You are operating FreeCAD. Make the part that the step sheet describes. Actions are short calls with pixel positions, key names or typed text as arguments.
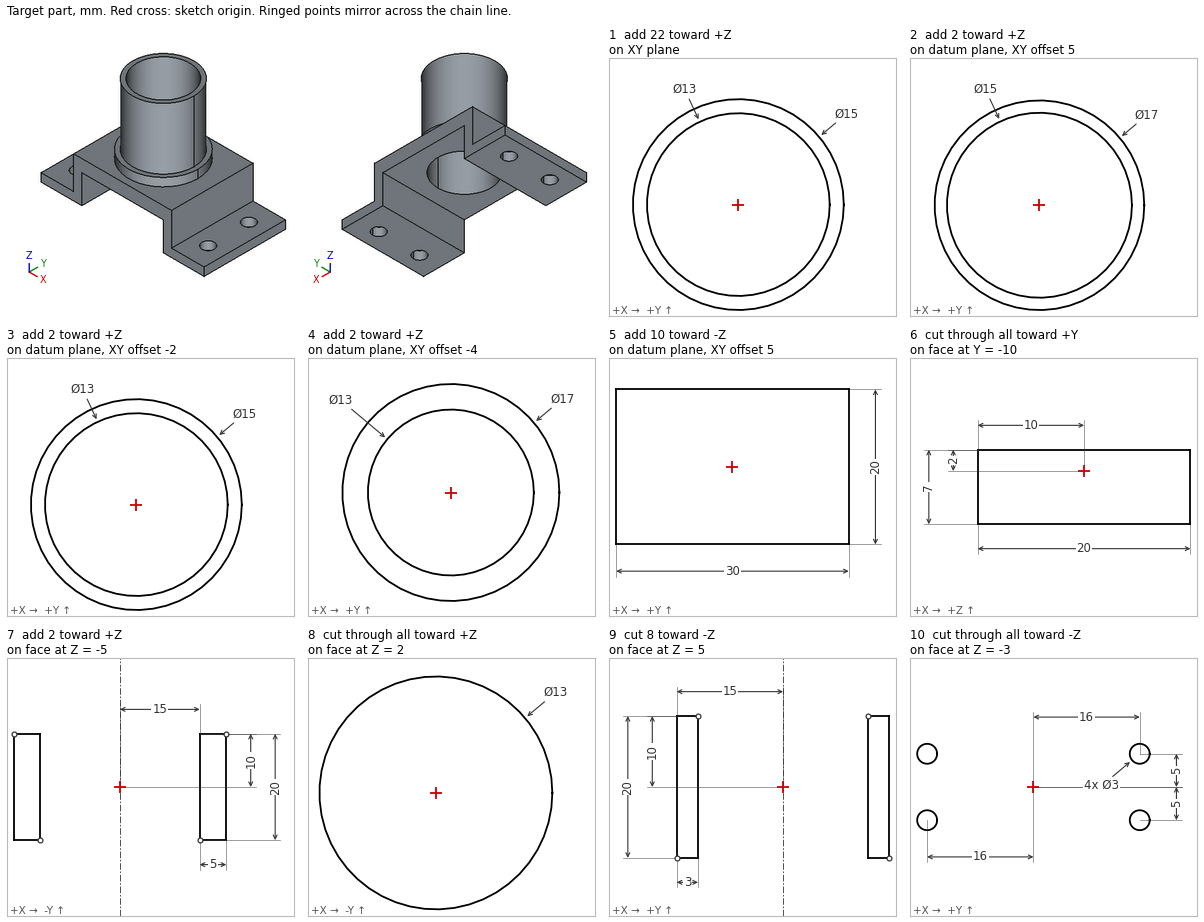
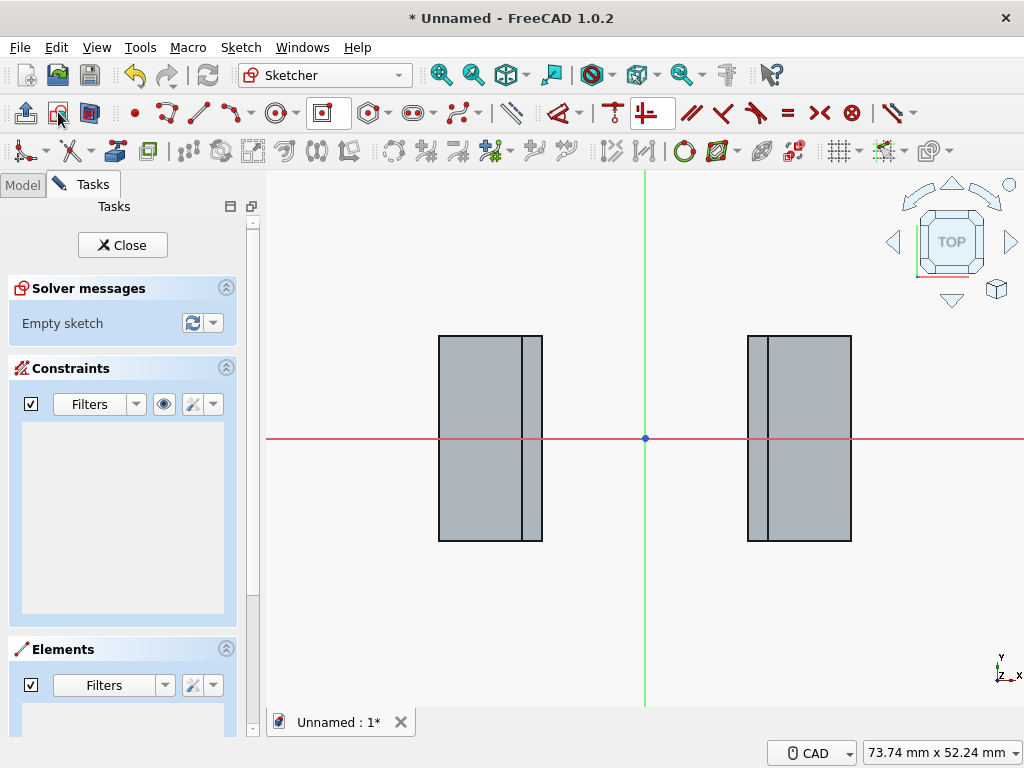
click(276, 114)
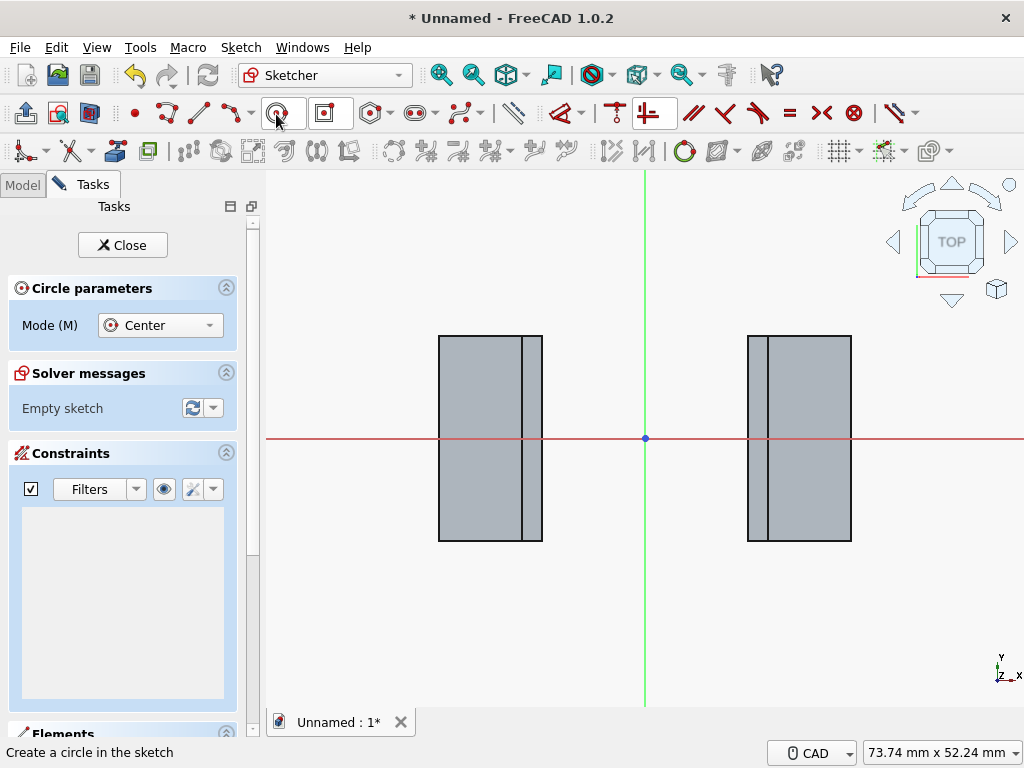
scroll(809, 387, up, 2)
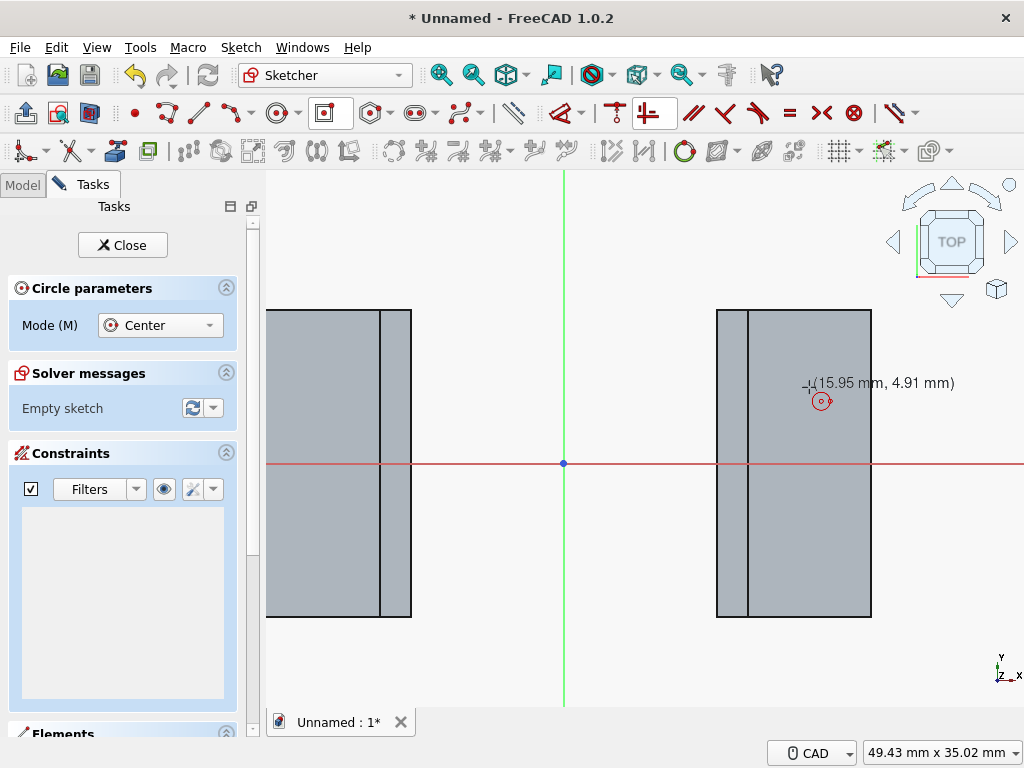
click(809, 387)
click(826, 371)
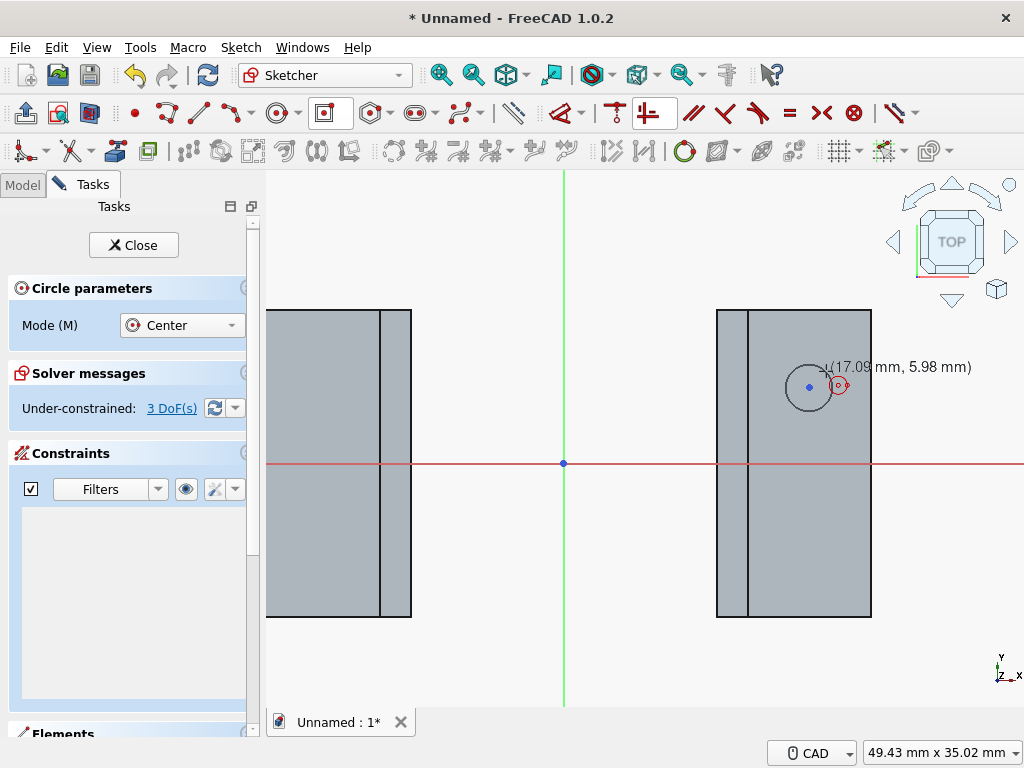
click(809, 540)
click(826, 524)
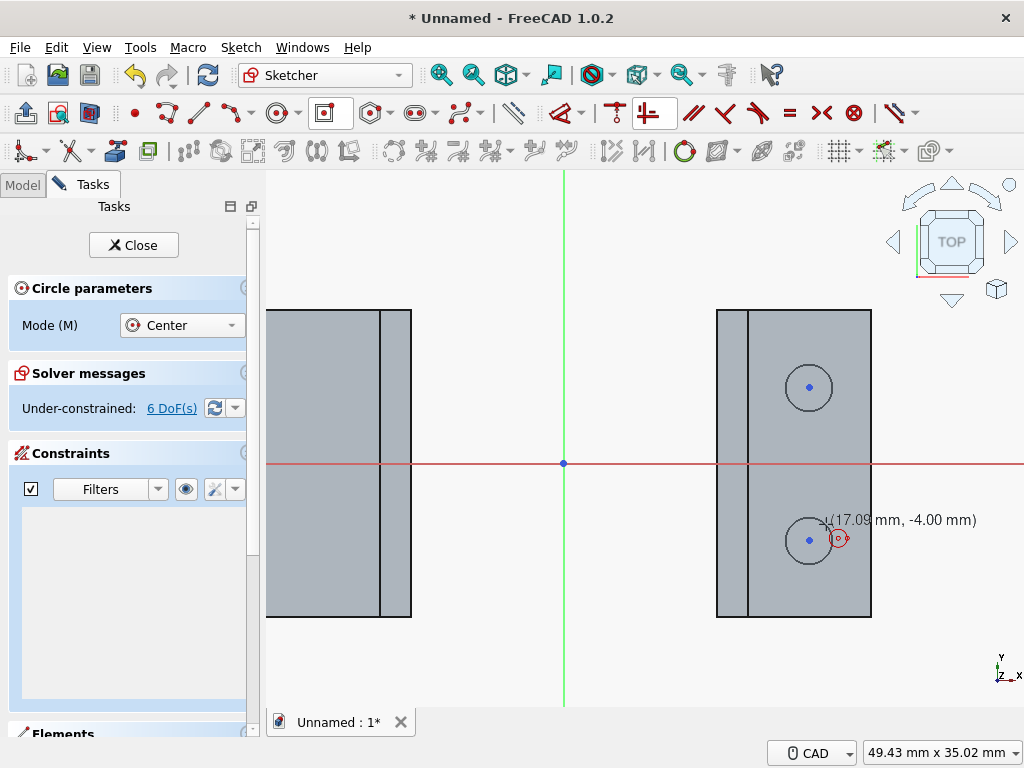
click(319, 540)
click(335, 524)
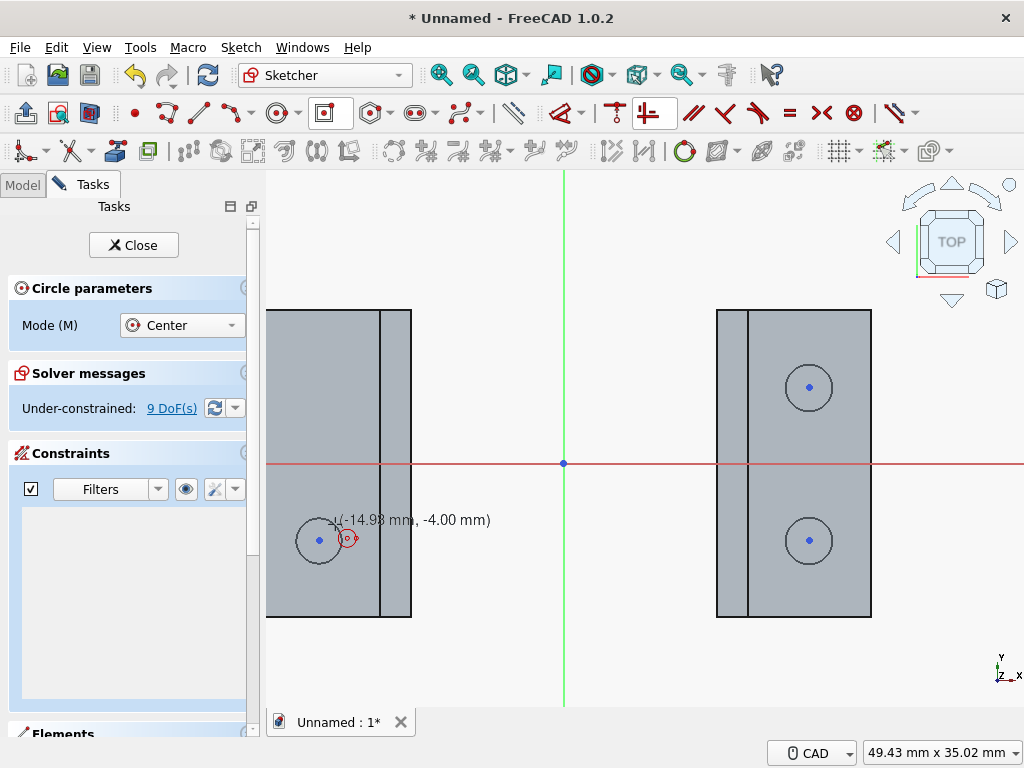
click(319, 387)
click(335, 371)
key(Escape)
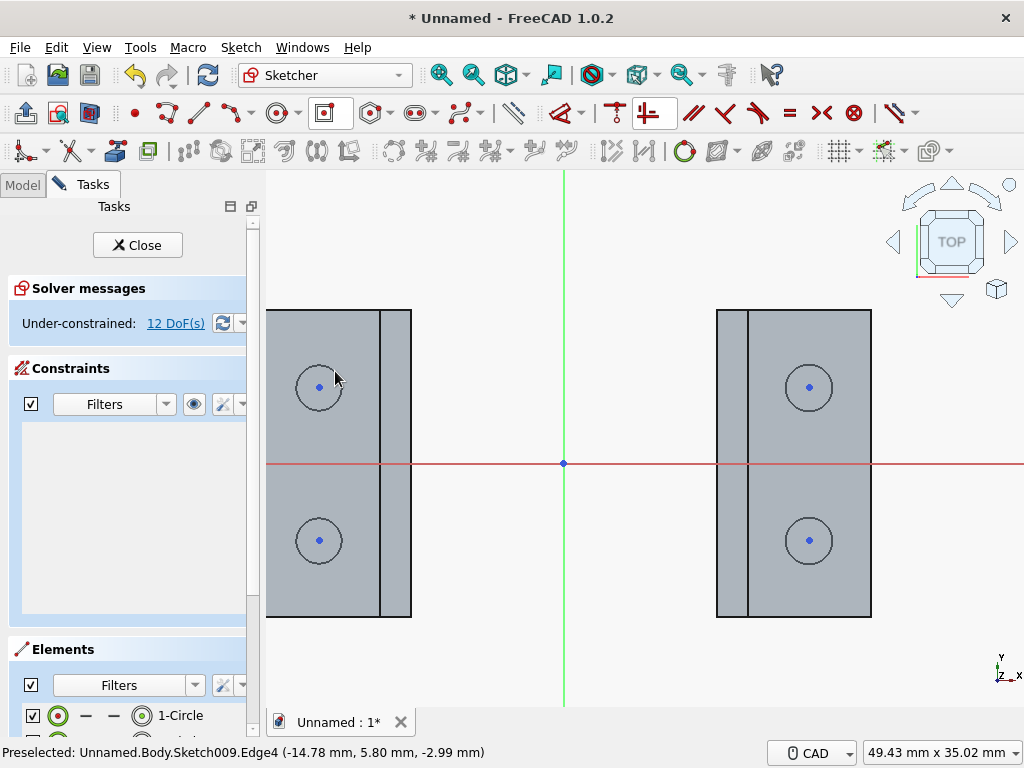
click(825, 371)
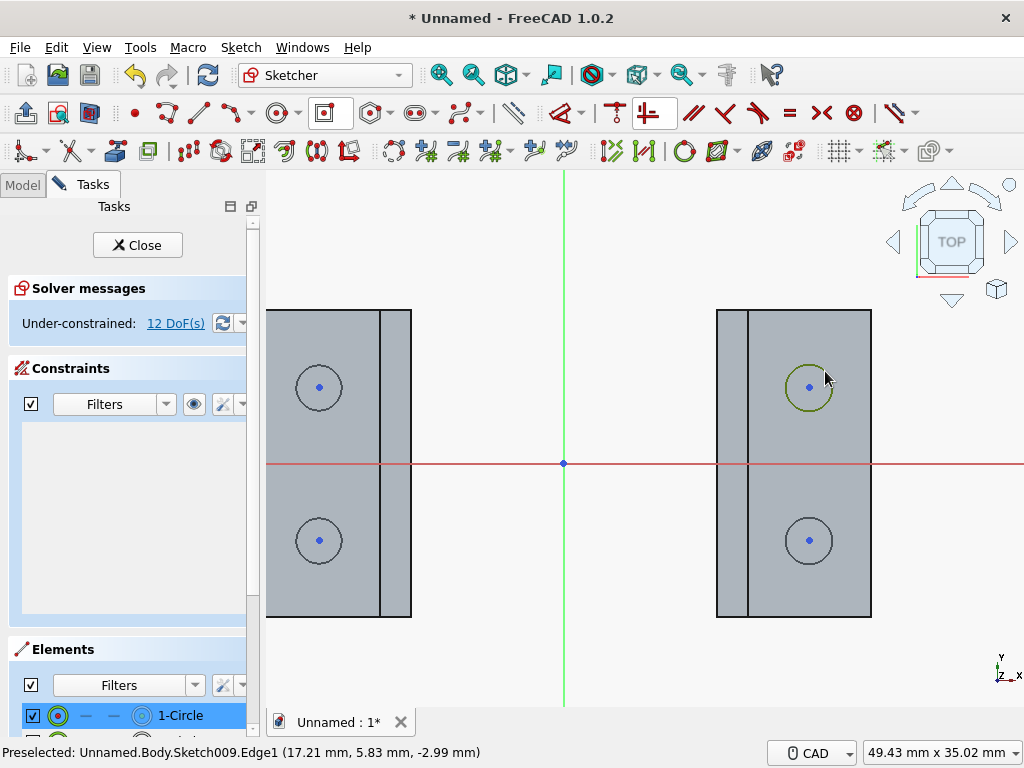
click(825, 524)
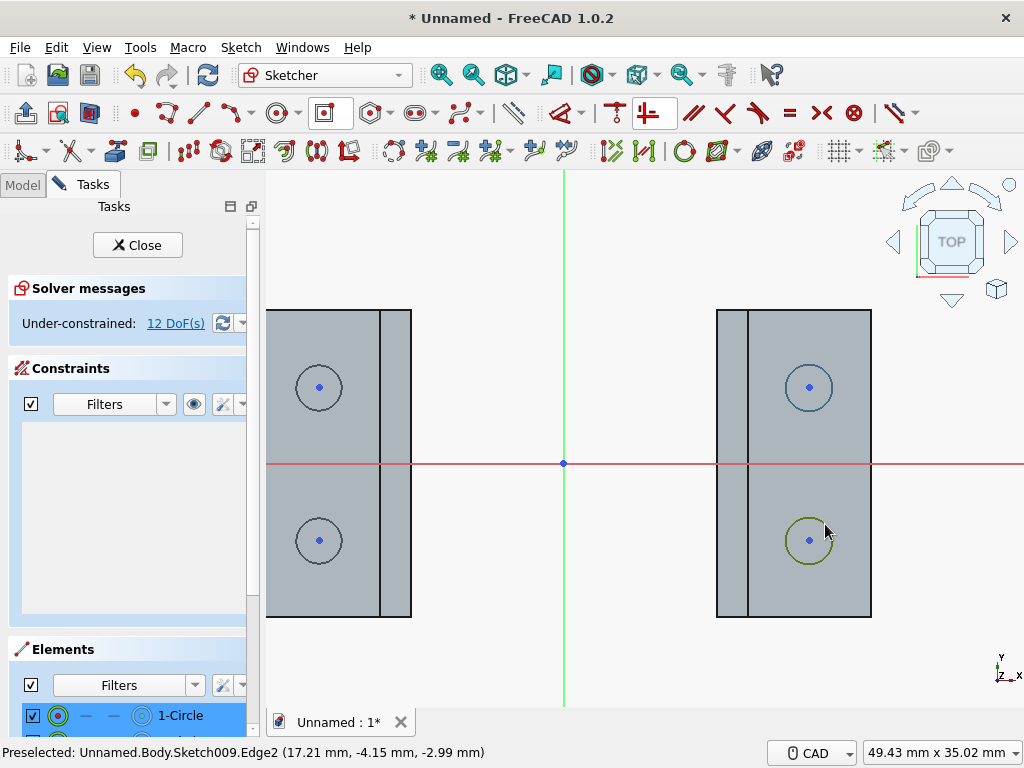
click(335, 525)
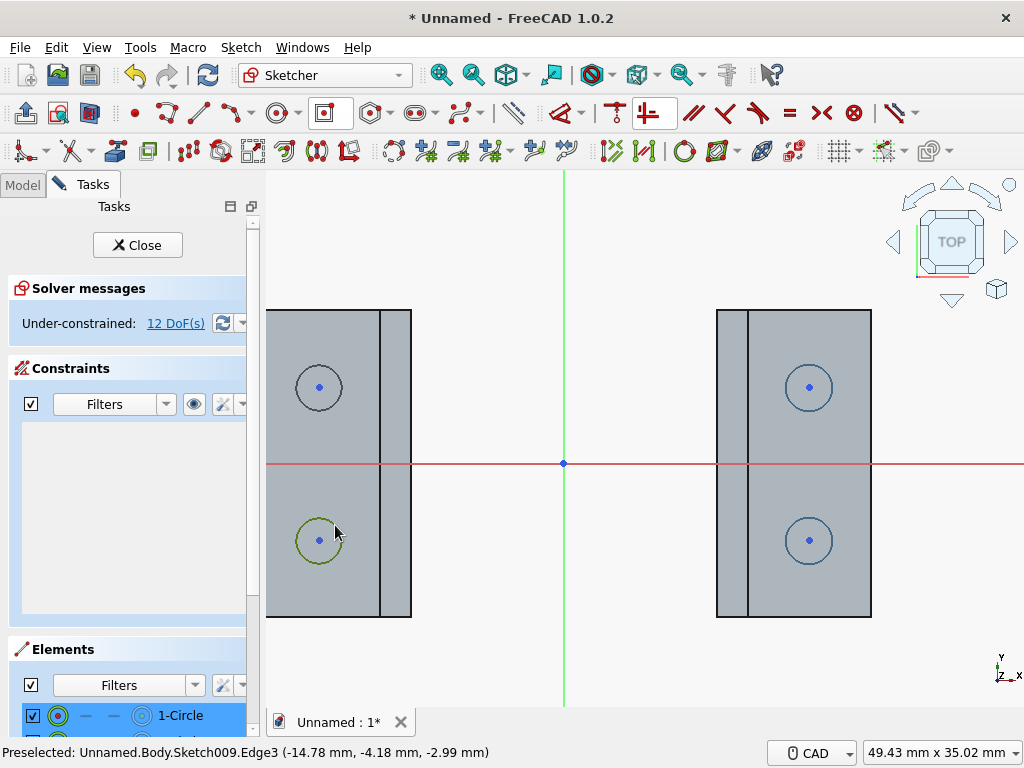
click(335, 372)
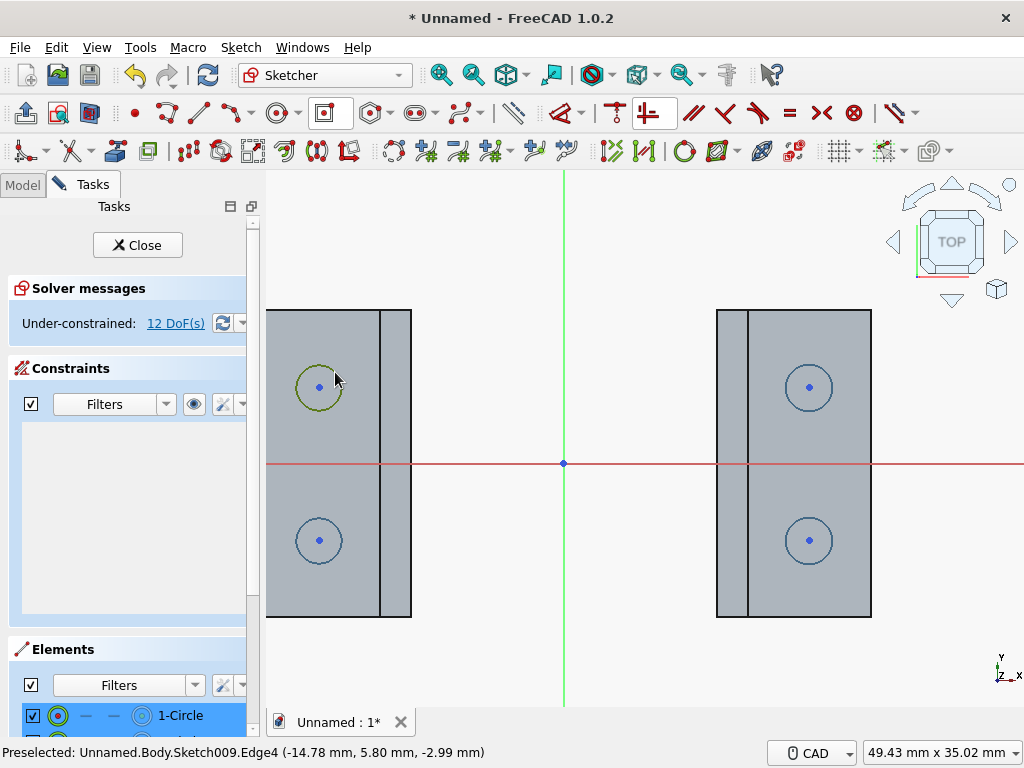
click(790, 114)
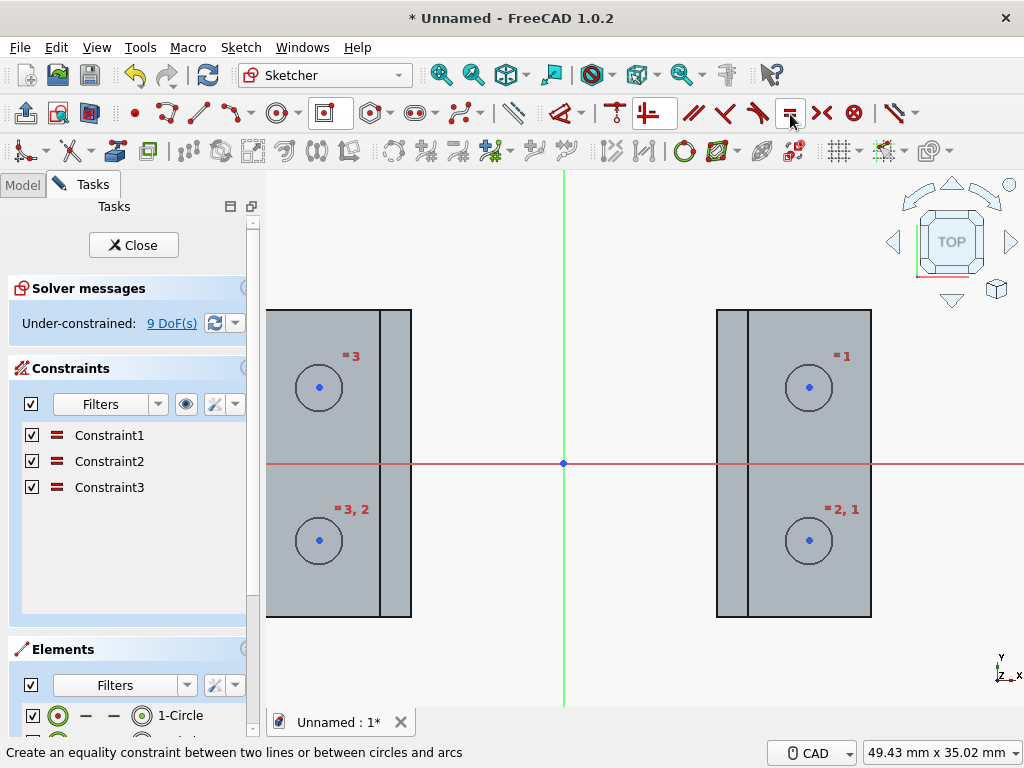
click(809, 388)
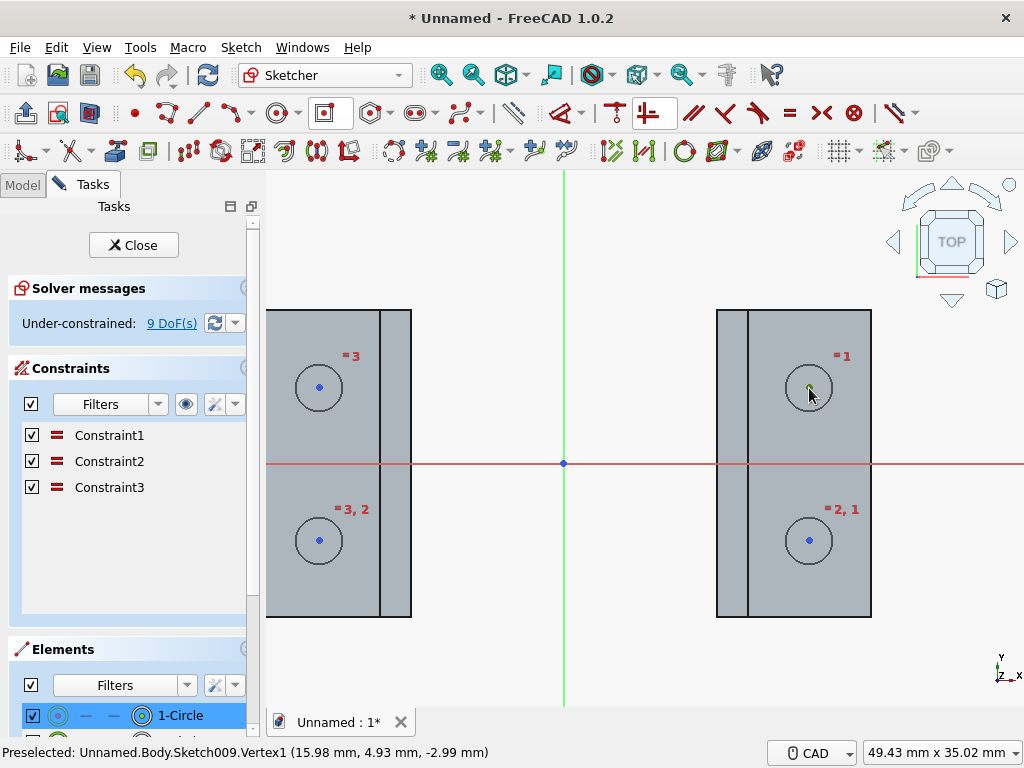
click(809, 541)